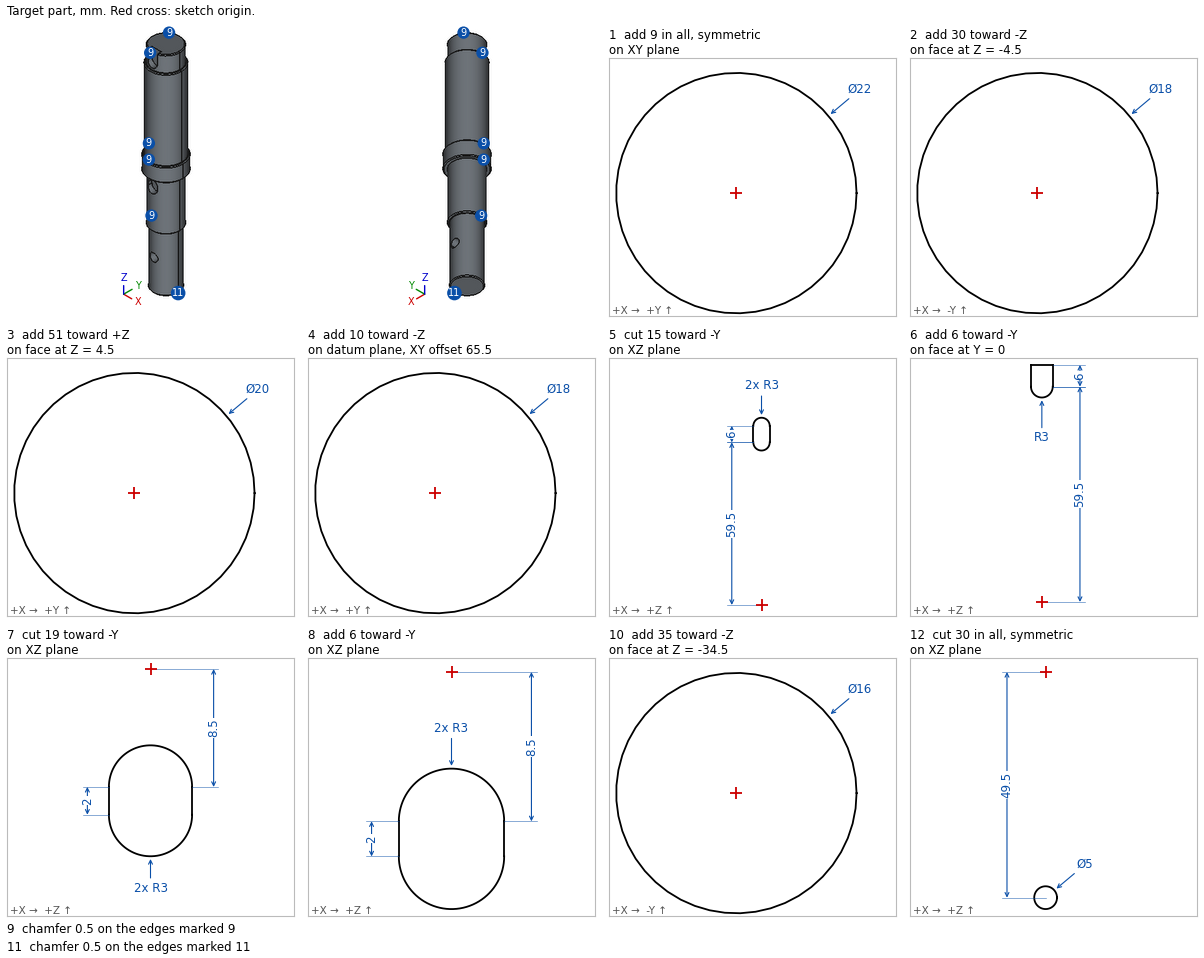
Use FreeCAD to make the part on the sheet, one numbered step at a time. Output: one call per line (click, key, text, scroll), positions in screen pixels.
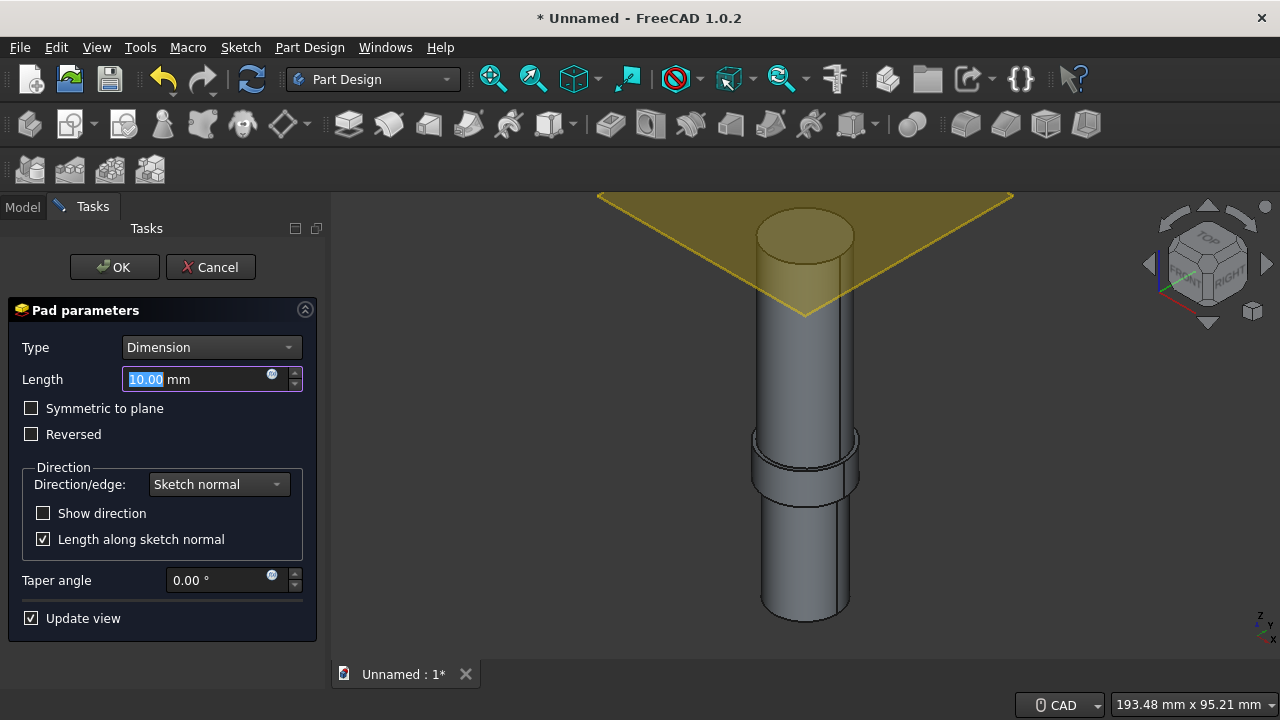
text(10)
key(Tab)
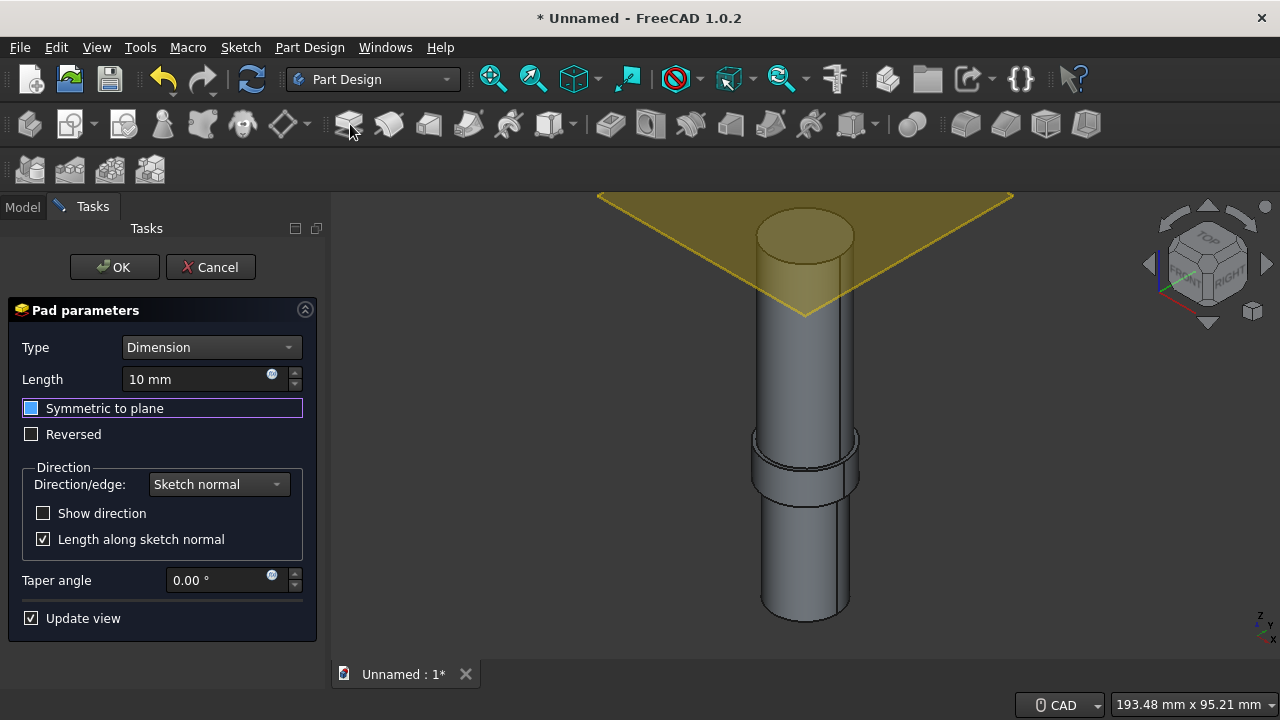
click(30, 434)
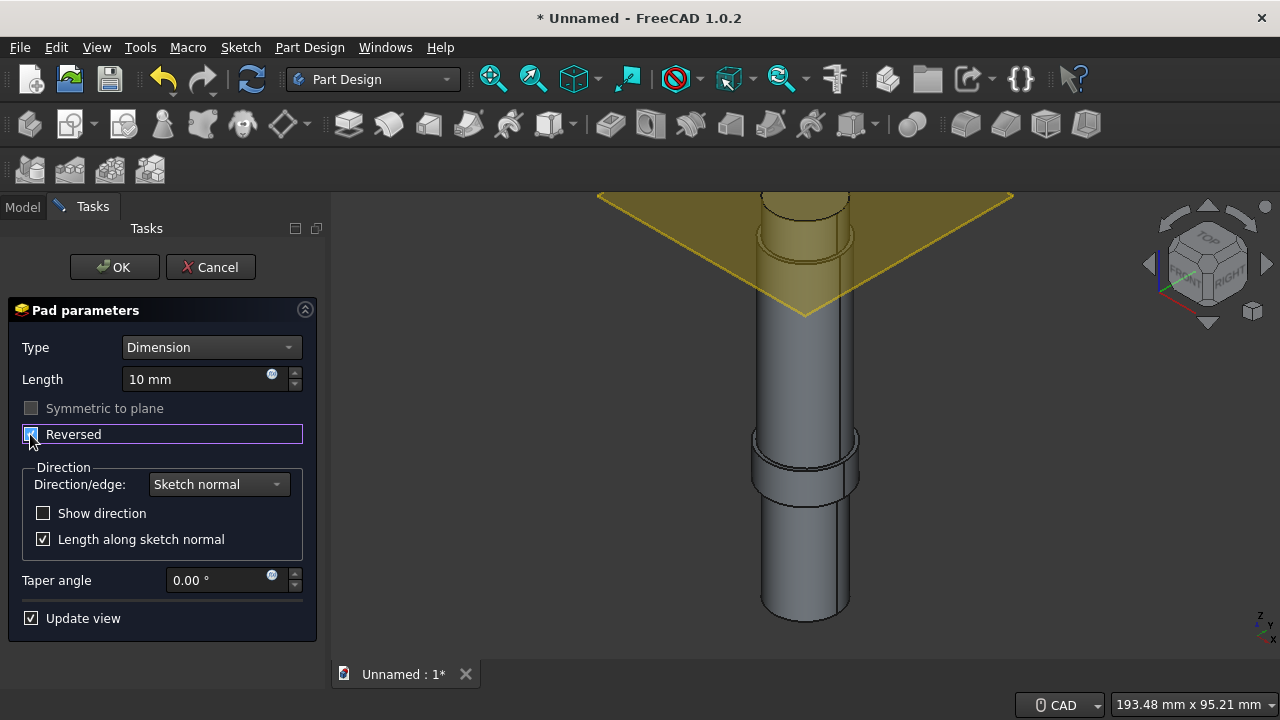
click(115, 267)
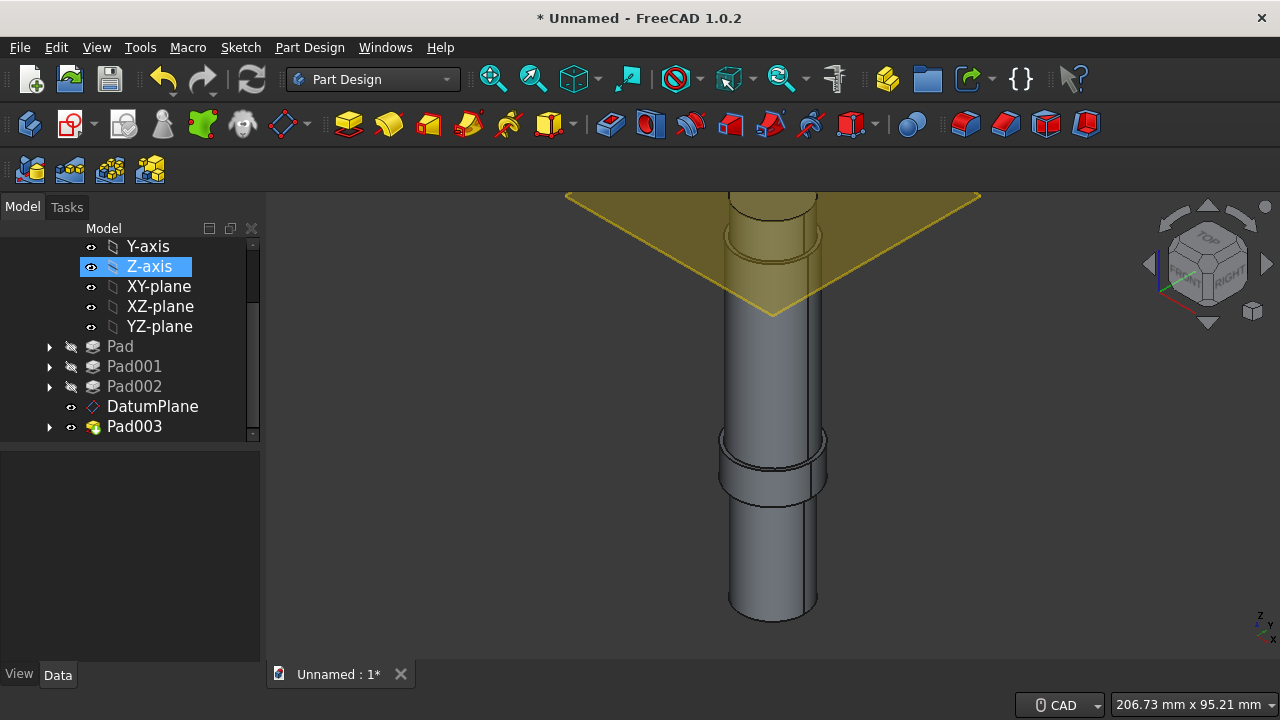
click(116, 407)
key(space)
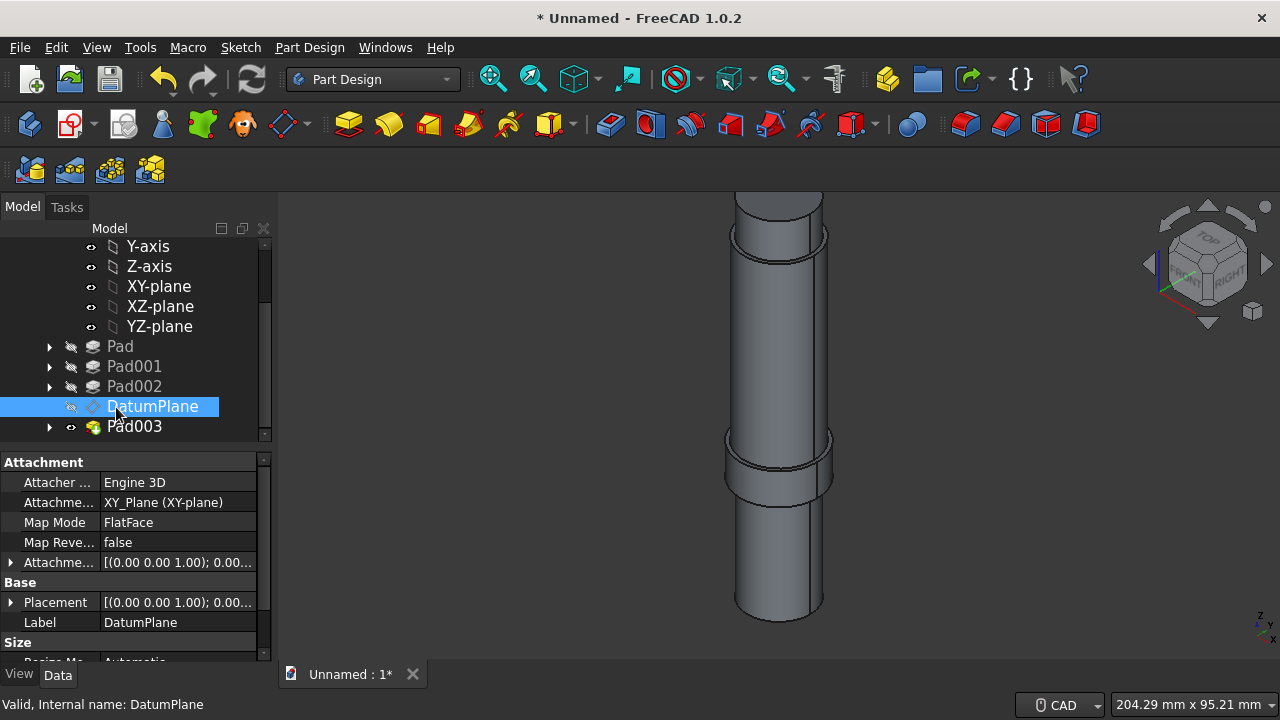
click(494, 80)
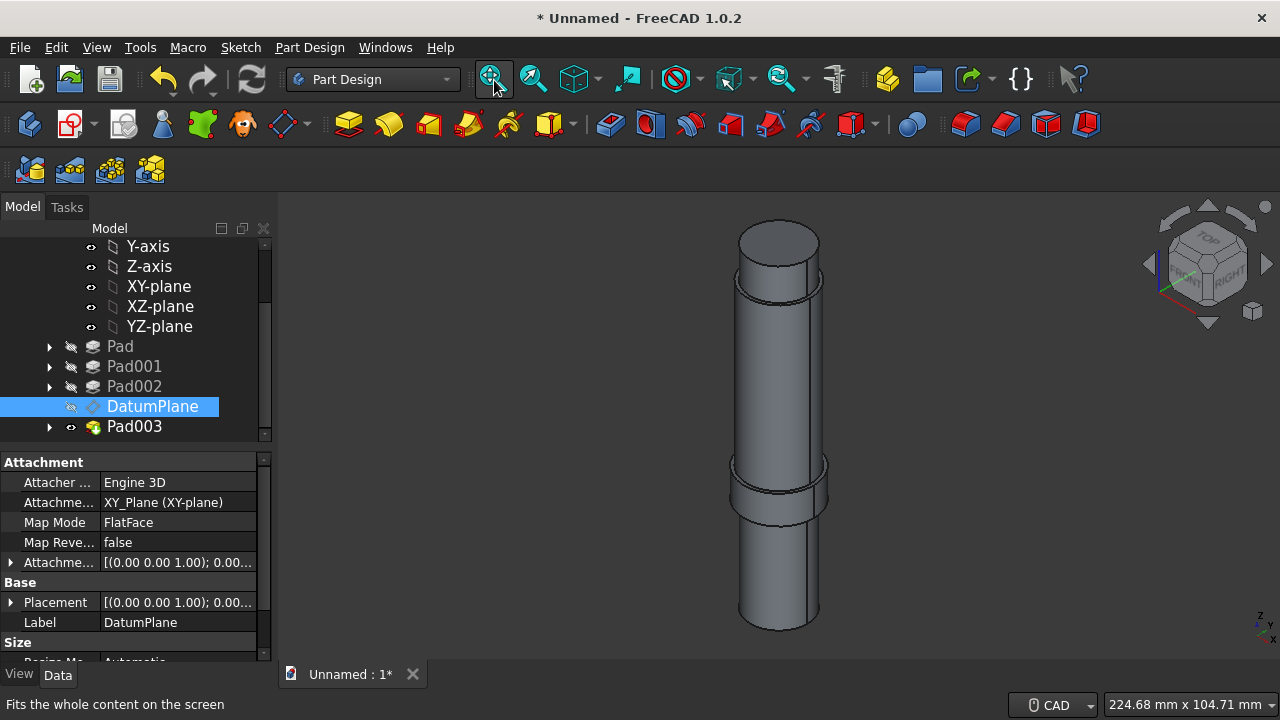
click(318, 619)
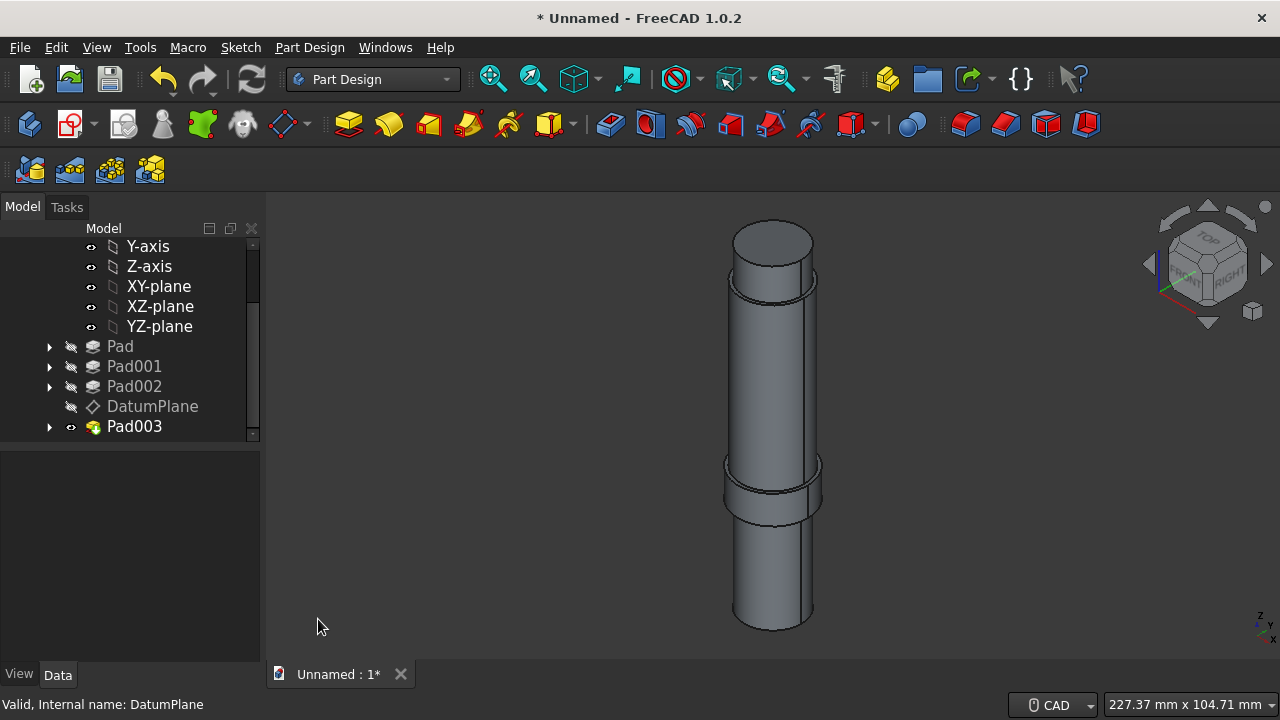
click(70, 124)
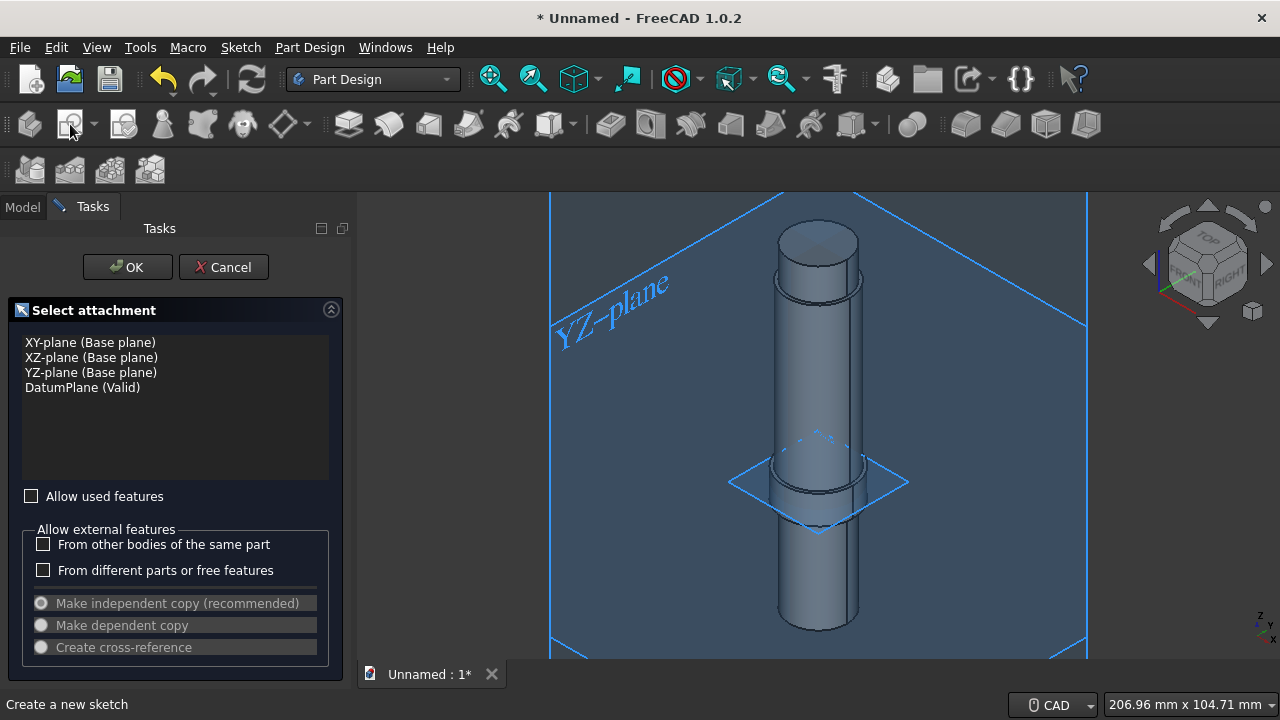
click(82, 358)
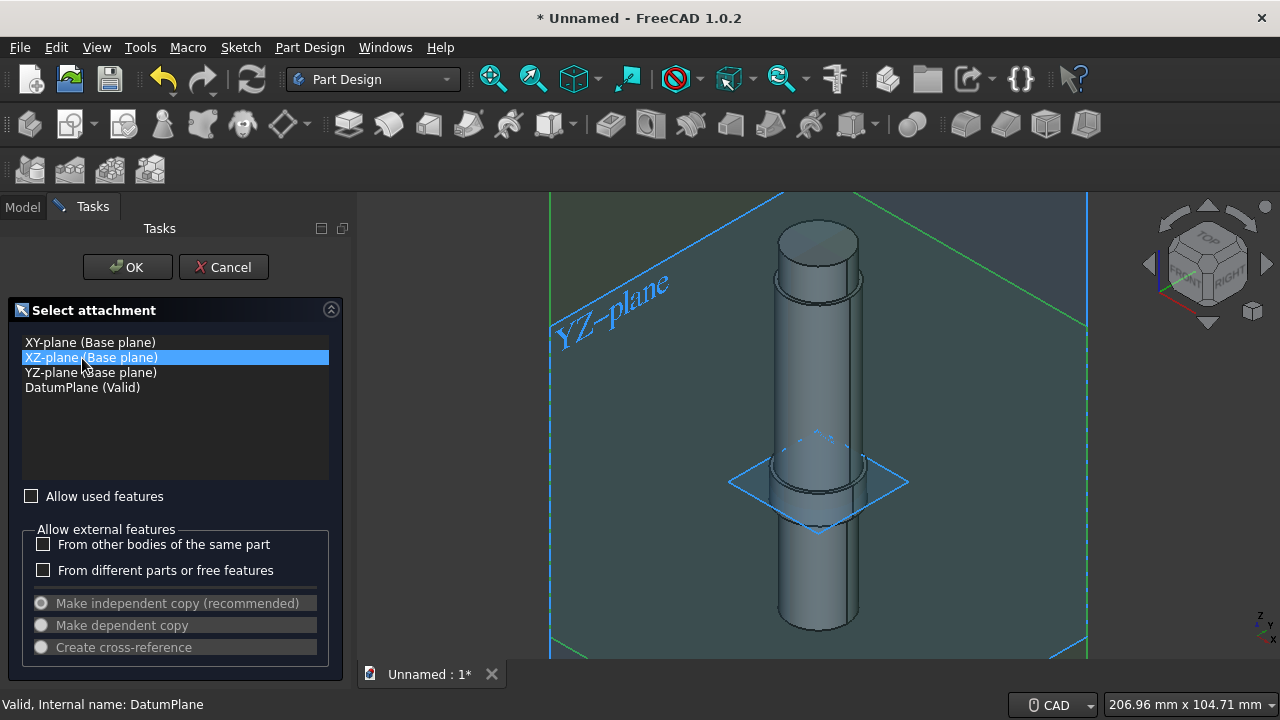
click(128, 267)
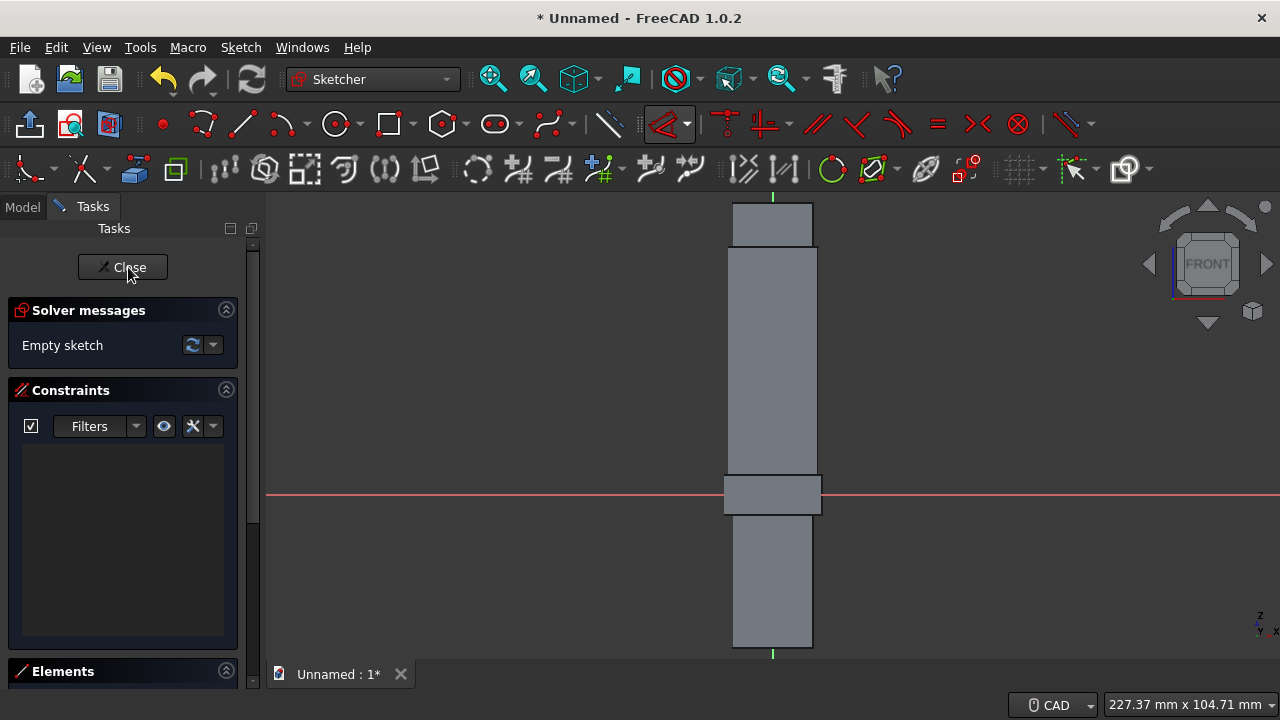
click(110, 124)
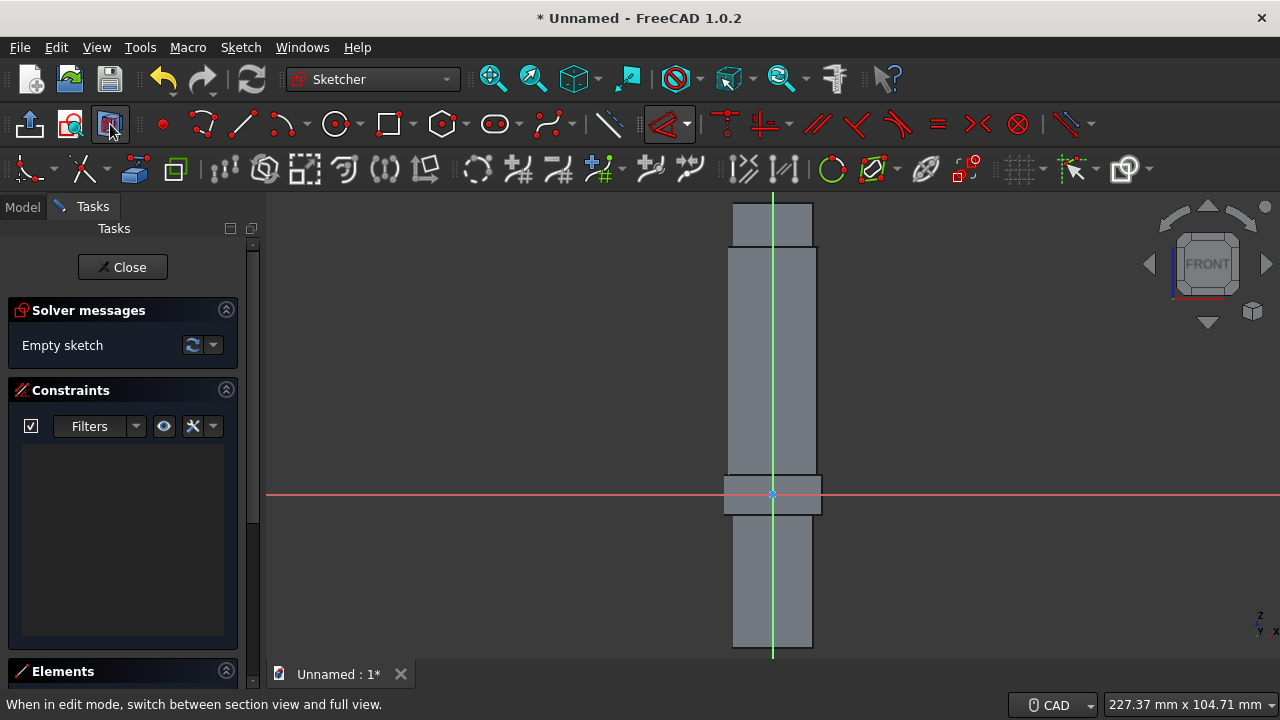
scroll(704, 426, down, 5)